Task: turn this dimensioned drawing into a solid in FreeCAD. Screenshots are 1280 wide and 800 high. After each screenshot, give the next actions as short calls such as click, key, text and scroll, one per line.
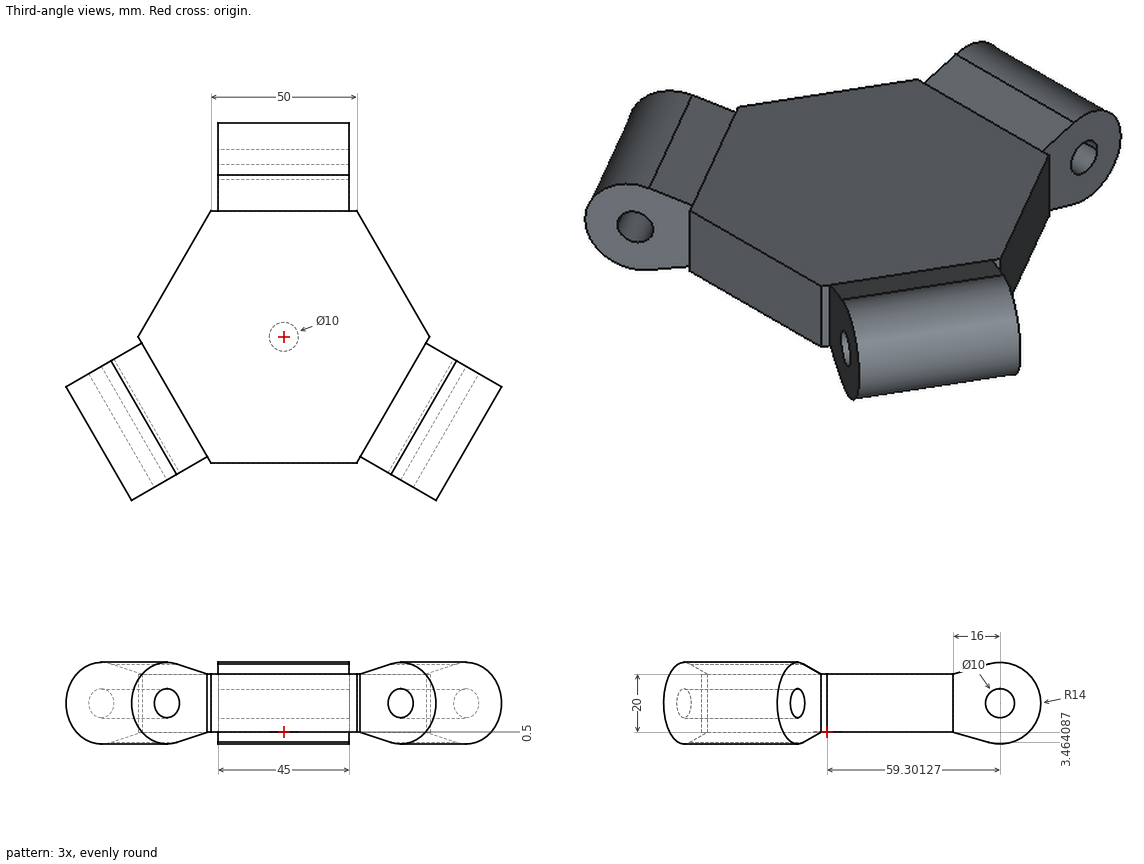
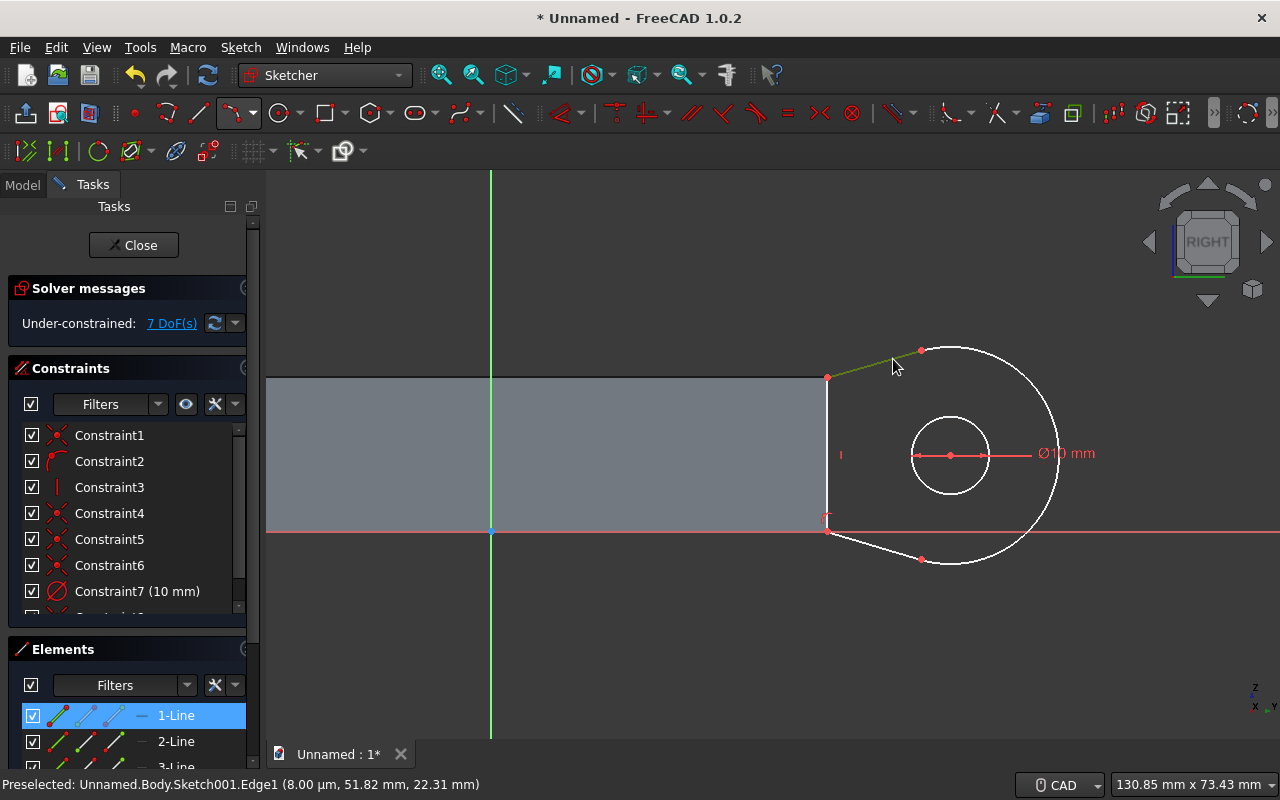
click(1031, 529)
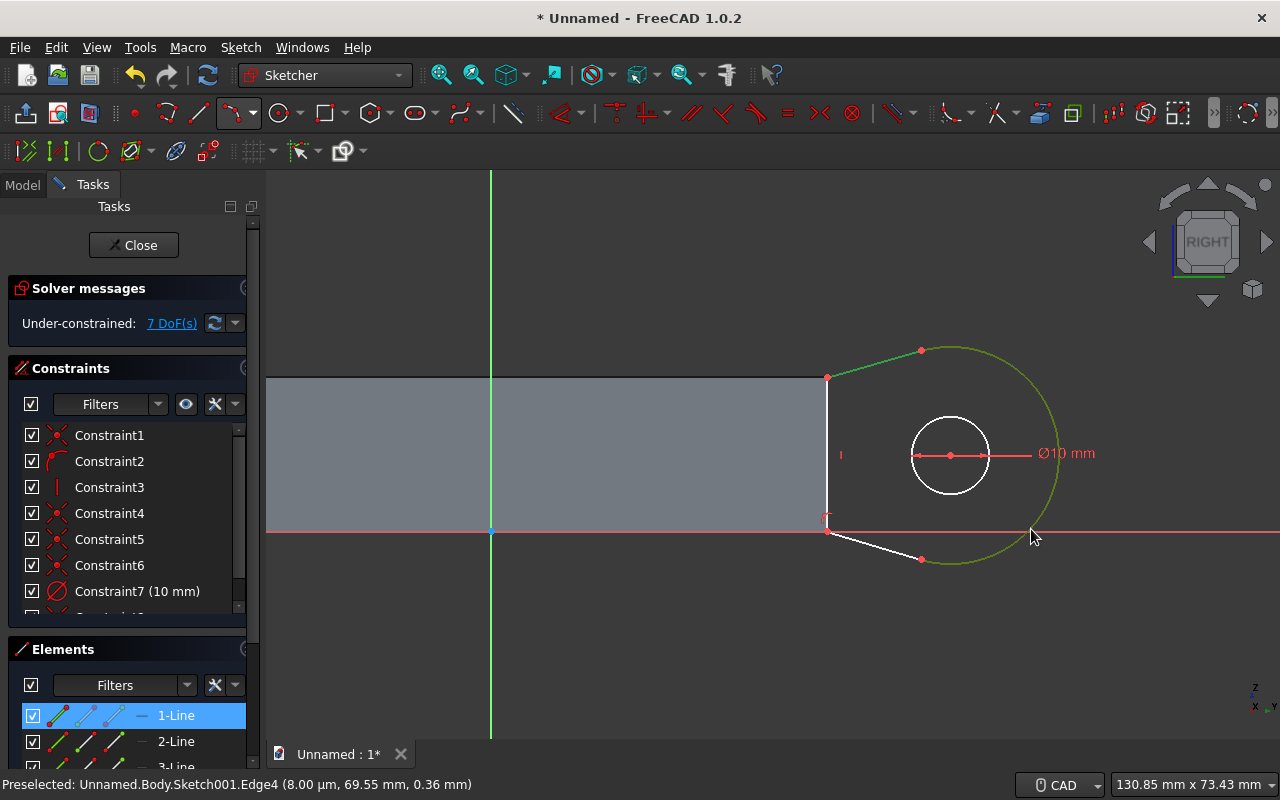
click(756, 114)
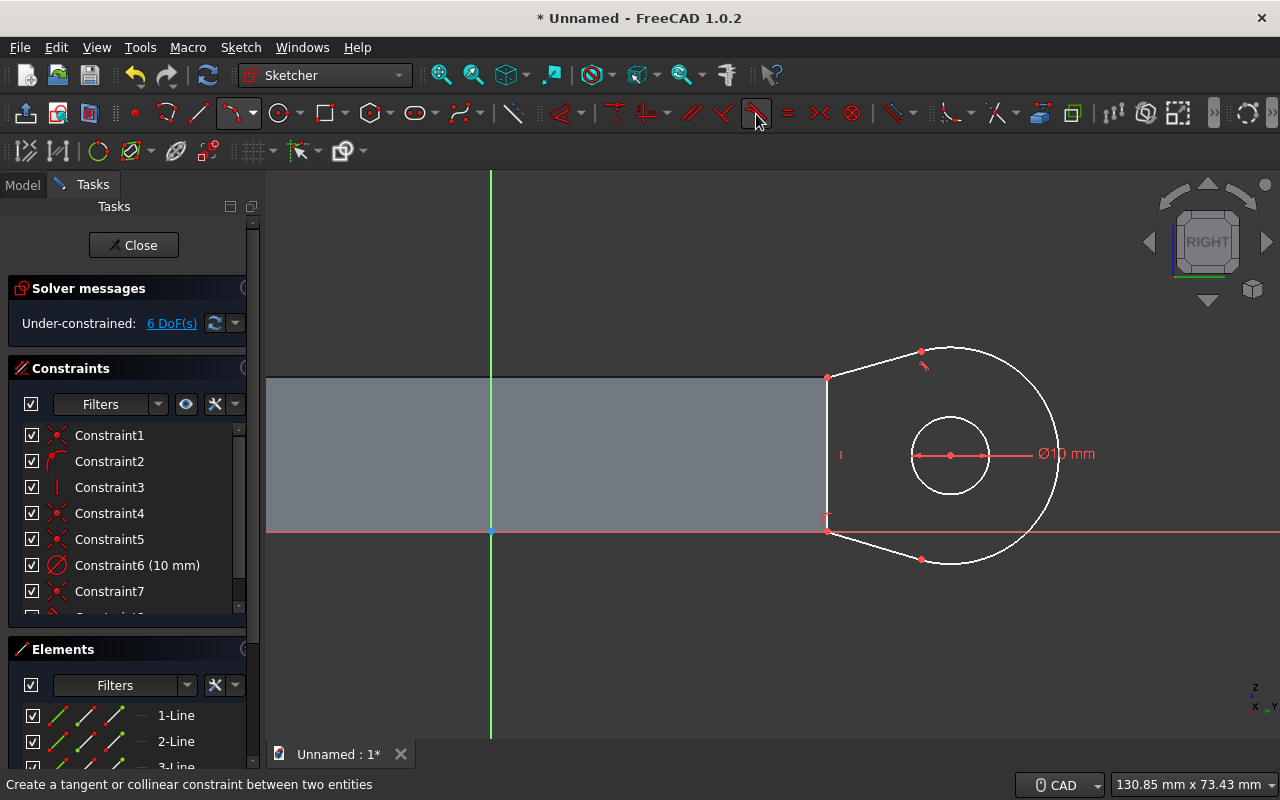
click(893, 552)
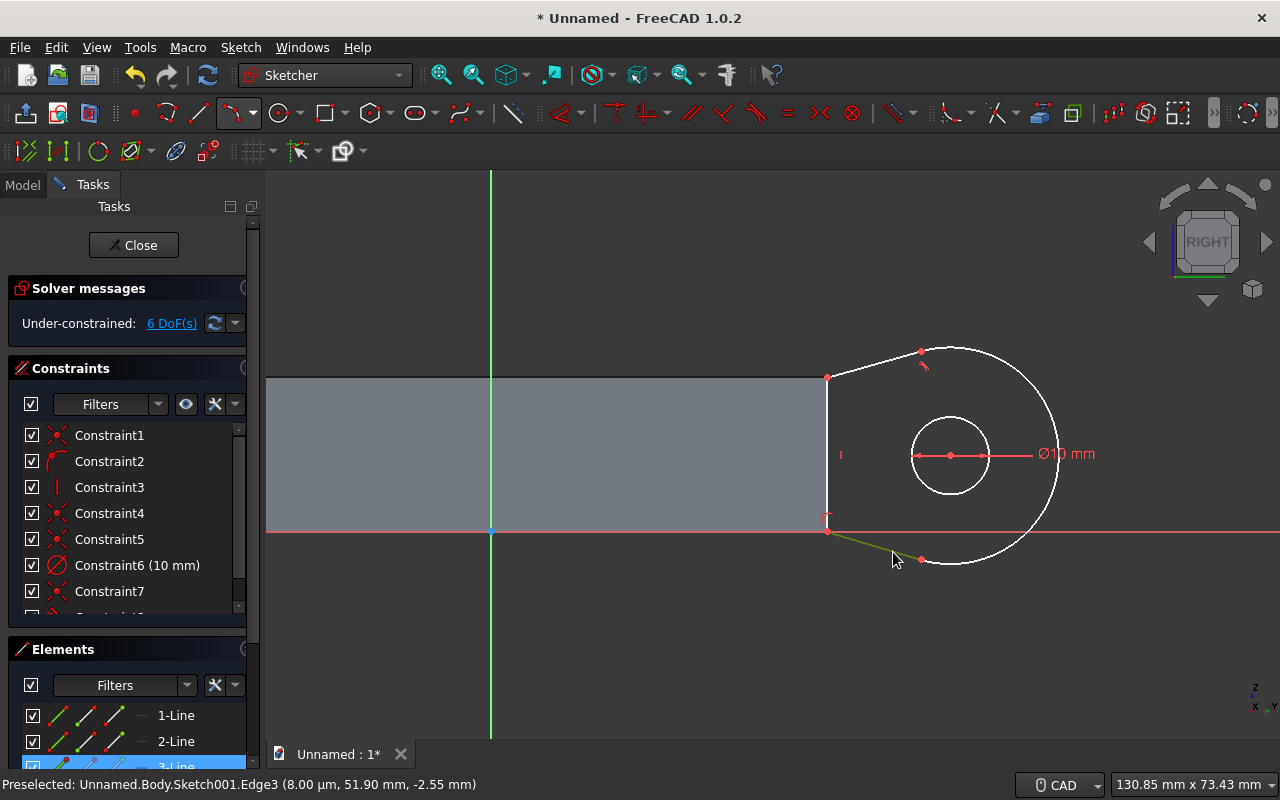
click(1031, 529)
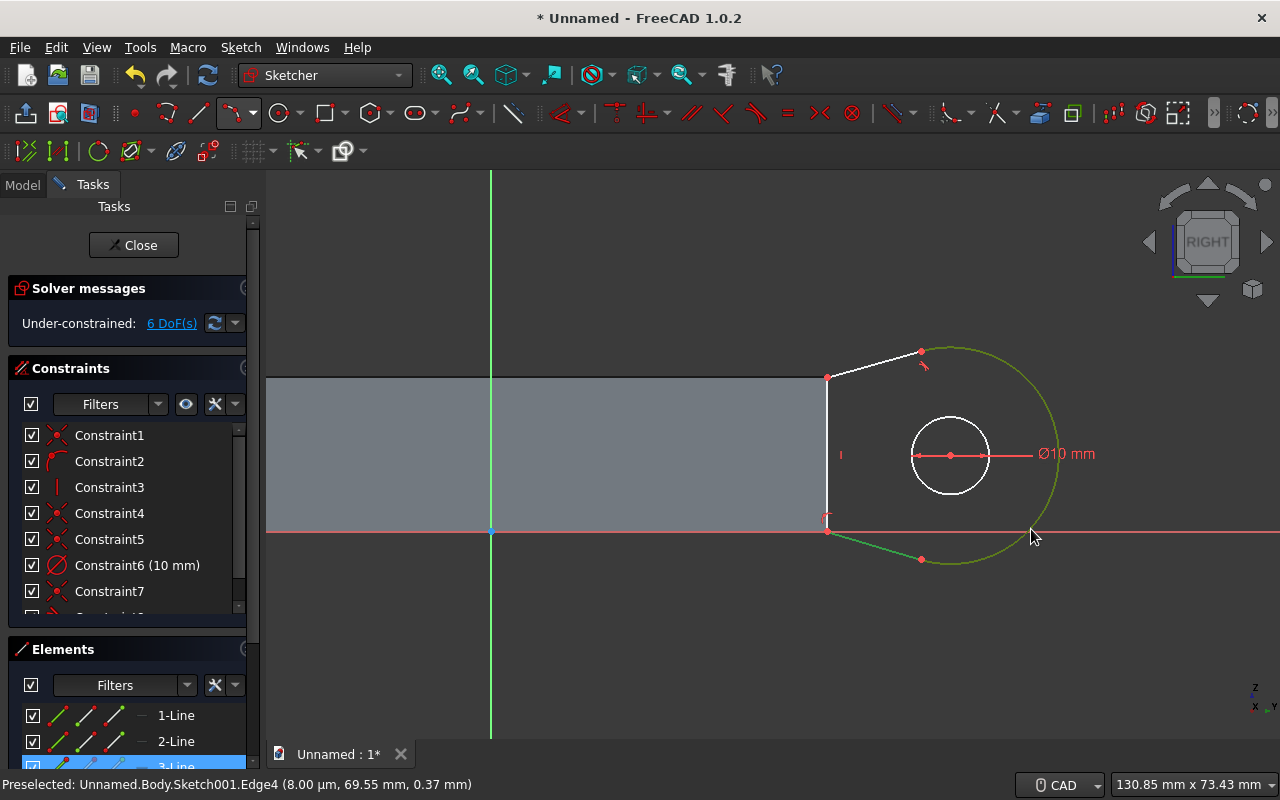
click(756, 114)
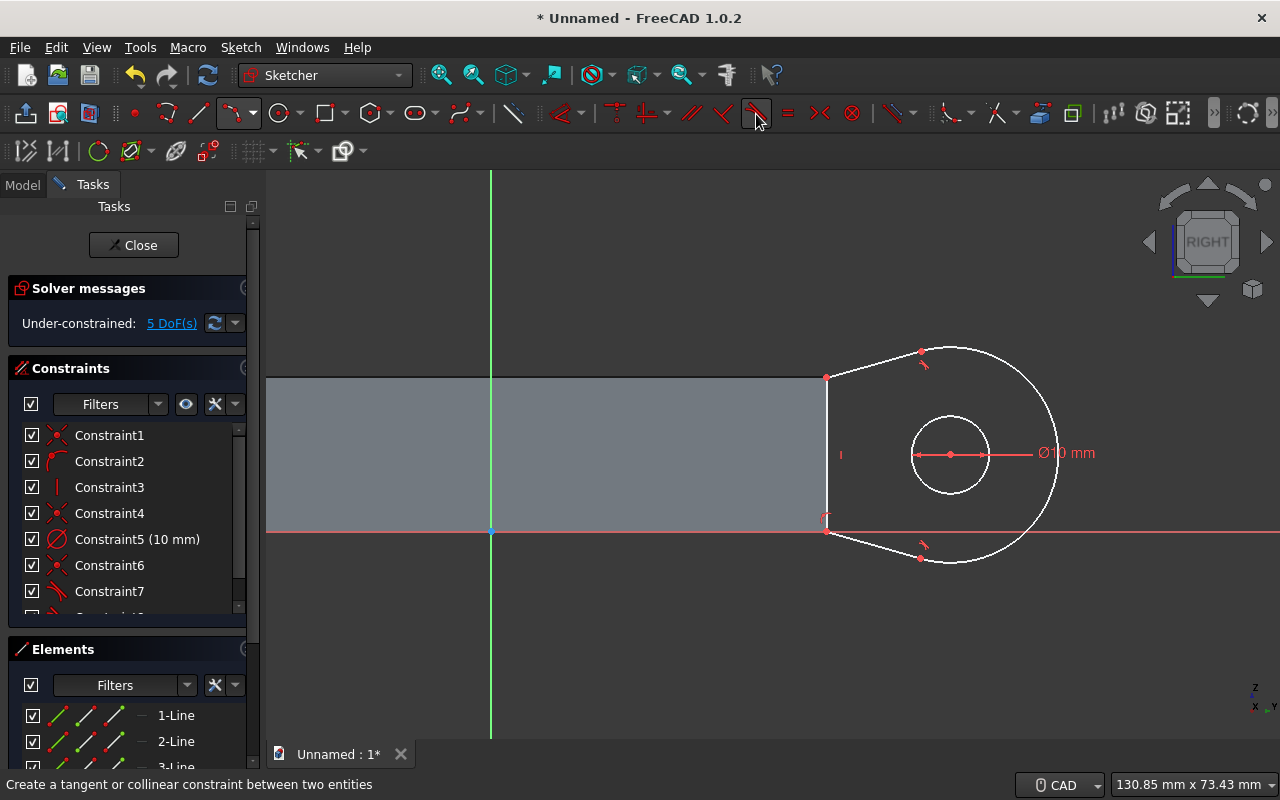
click(560, 114)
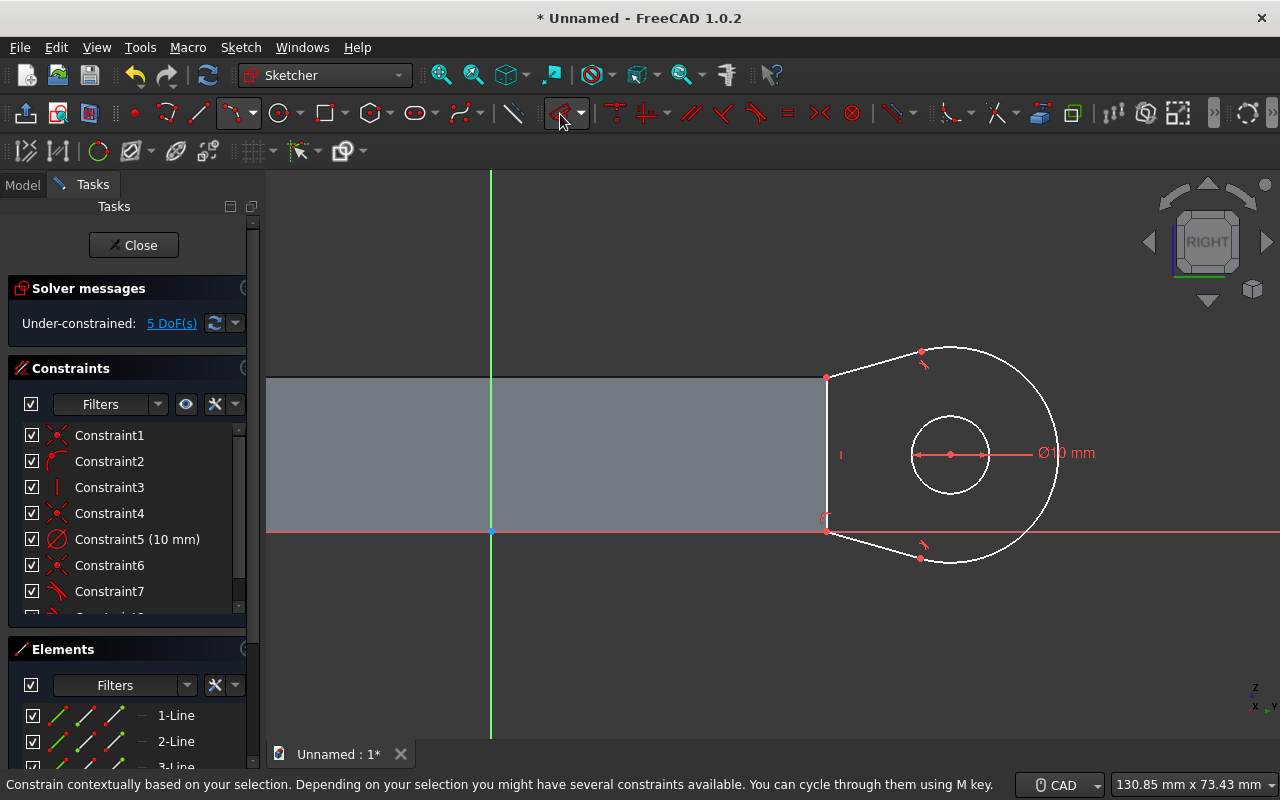
click(1030, 382)
click(1054, 360)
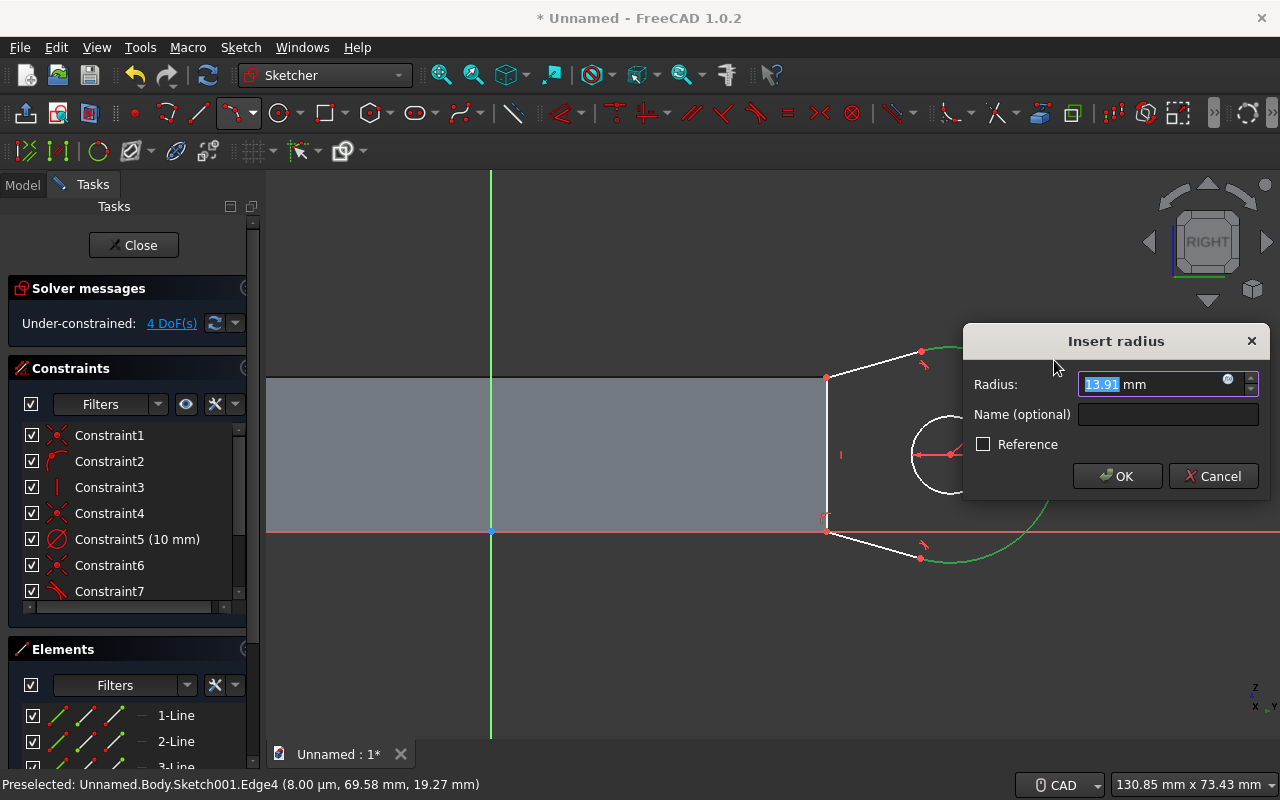
text(14)
key(Return)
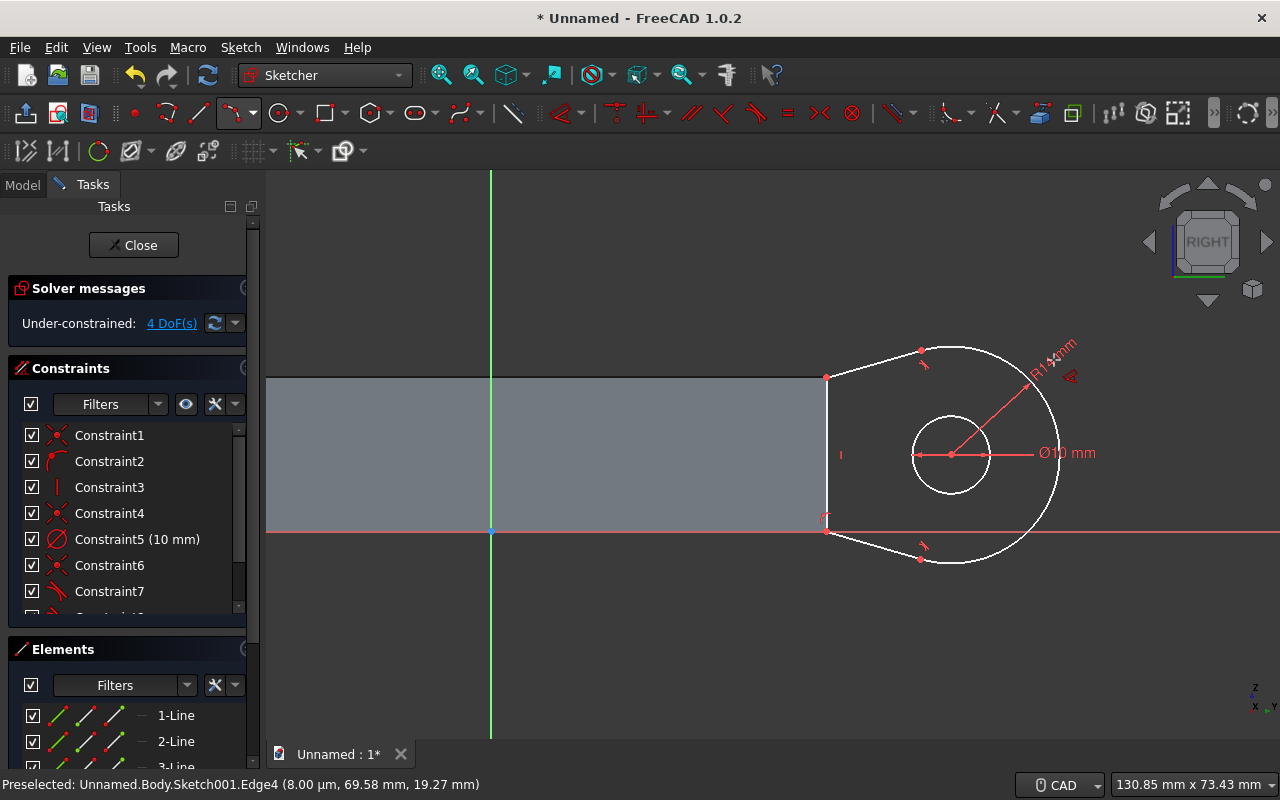
click(827, 424)
click(861, 455)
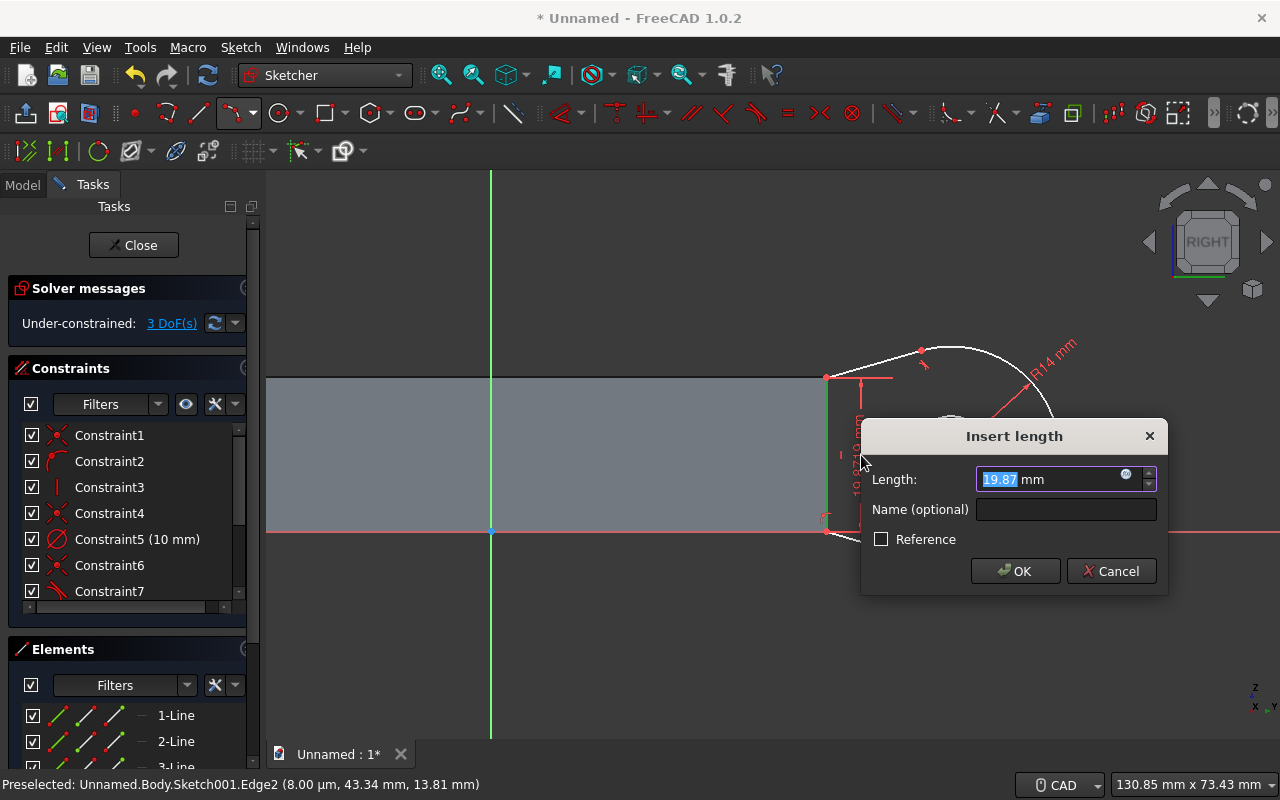
text(20)
key(Return)